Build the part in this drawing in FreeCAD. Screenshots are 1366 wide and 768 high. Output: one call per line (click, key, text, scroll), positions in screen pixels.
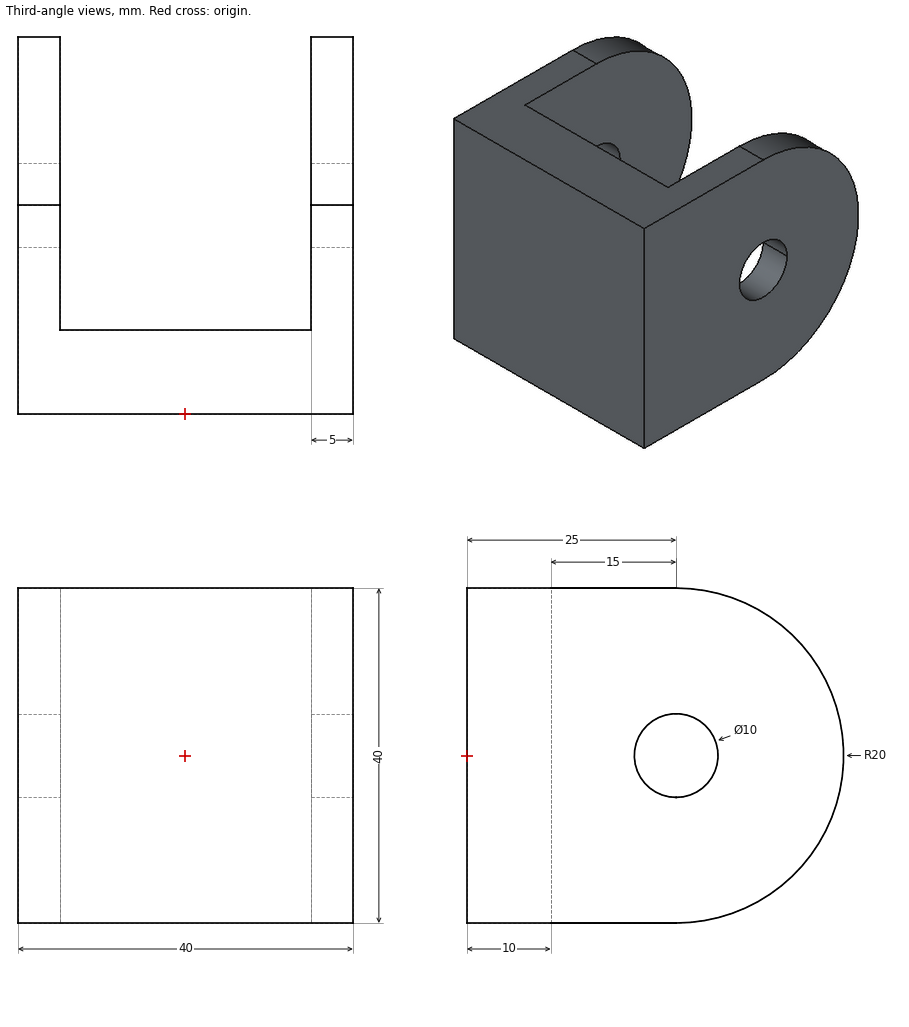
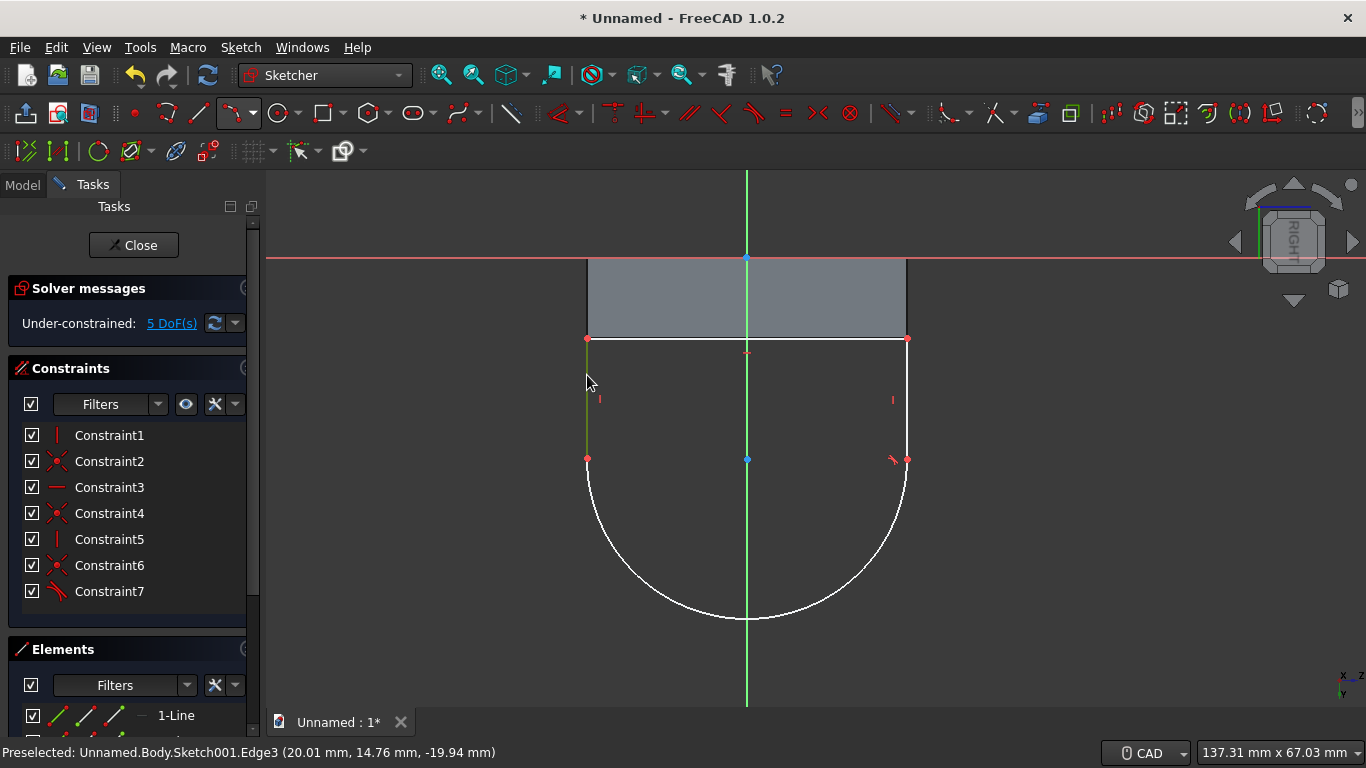
click(653, 588)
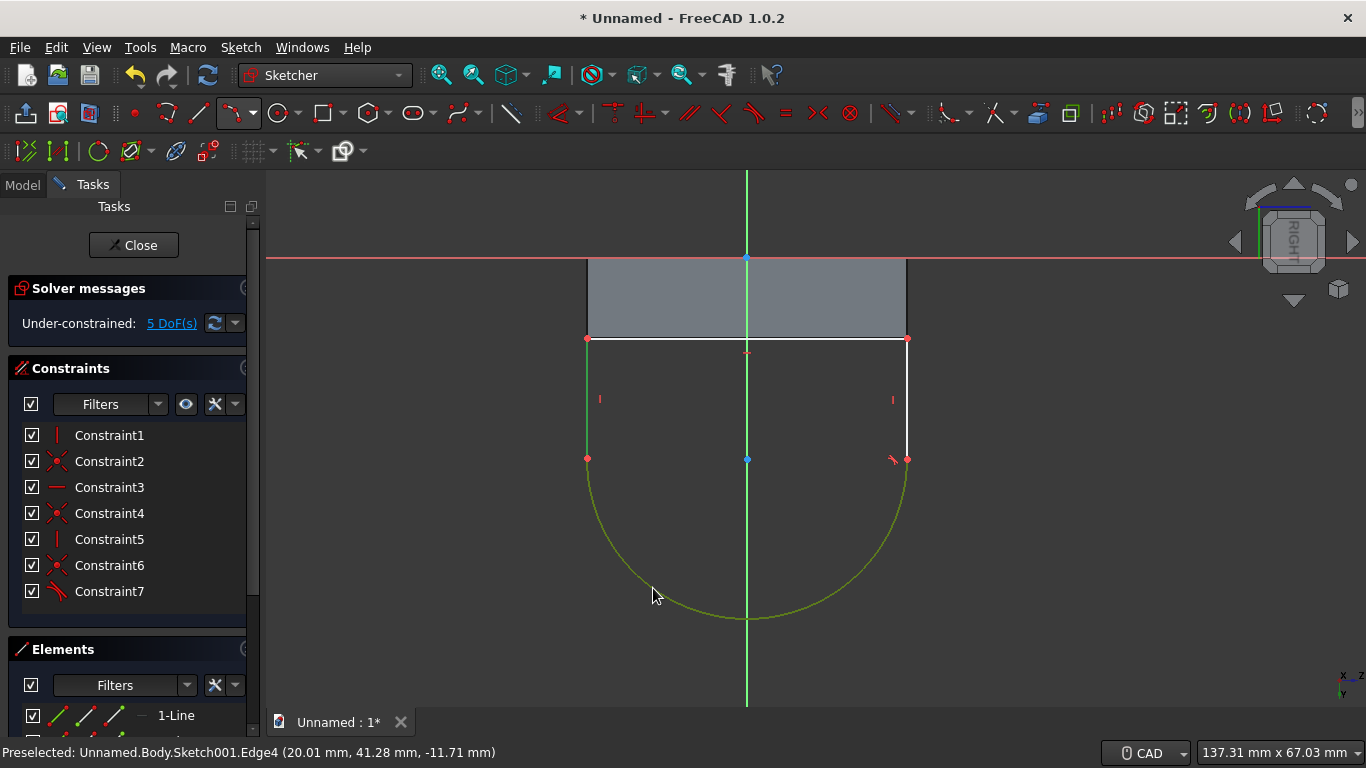
key(t)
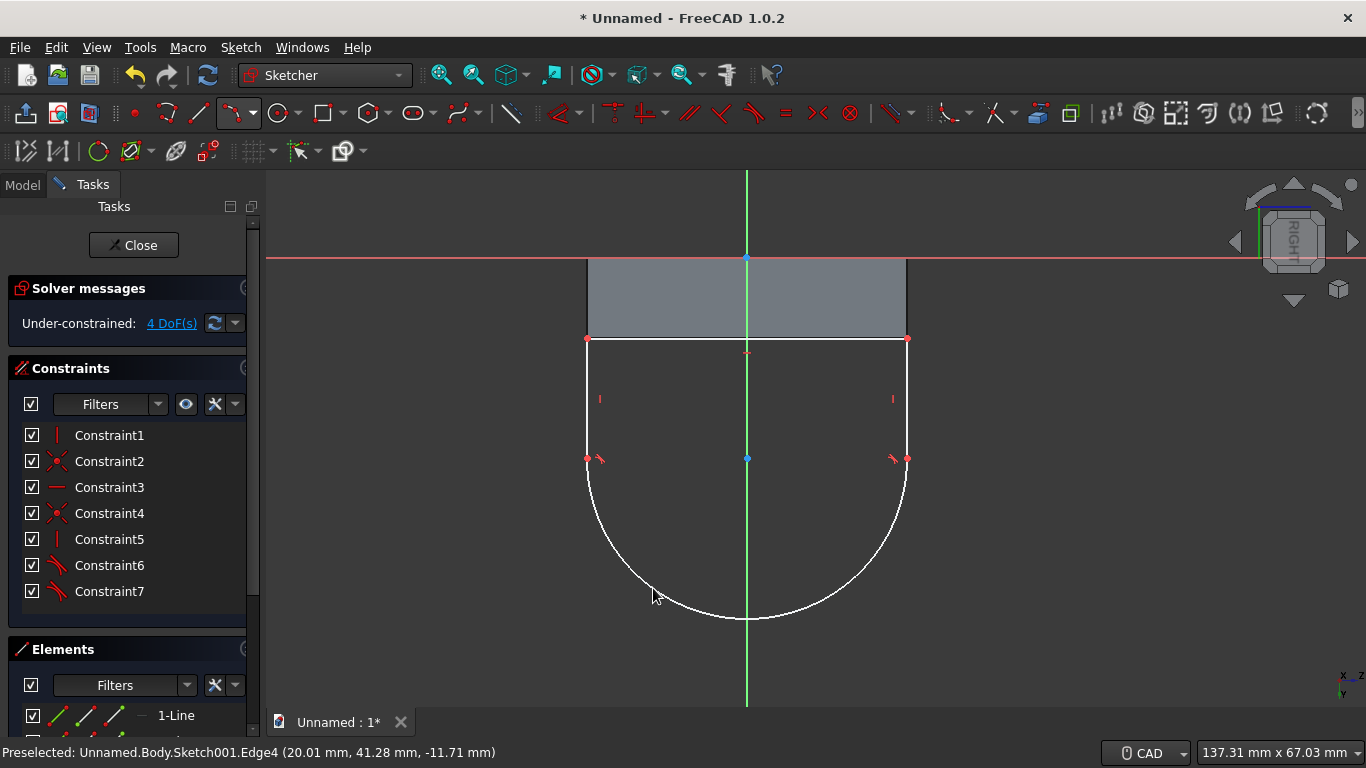
click(747, 459)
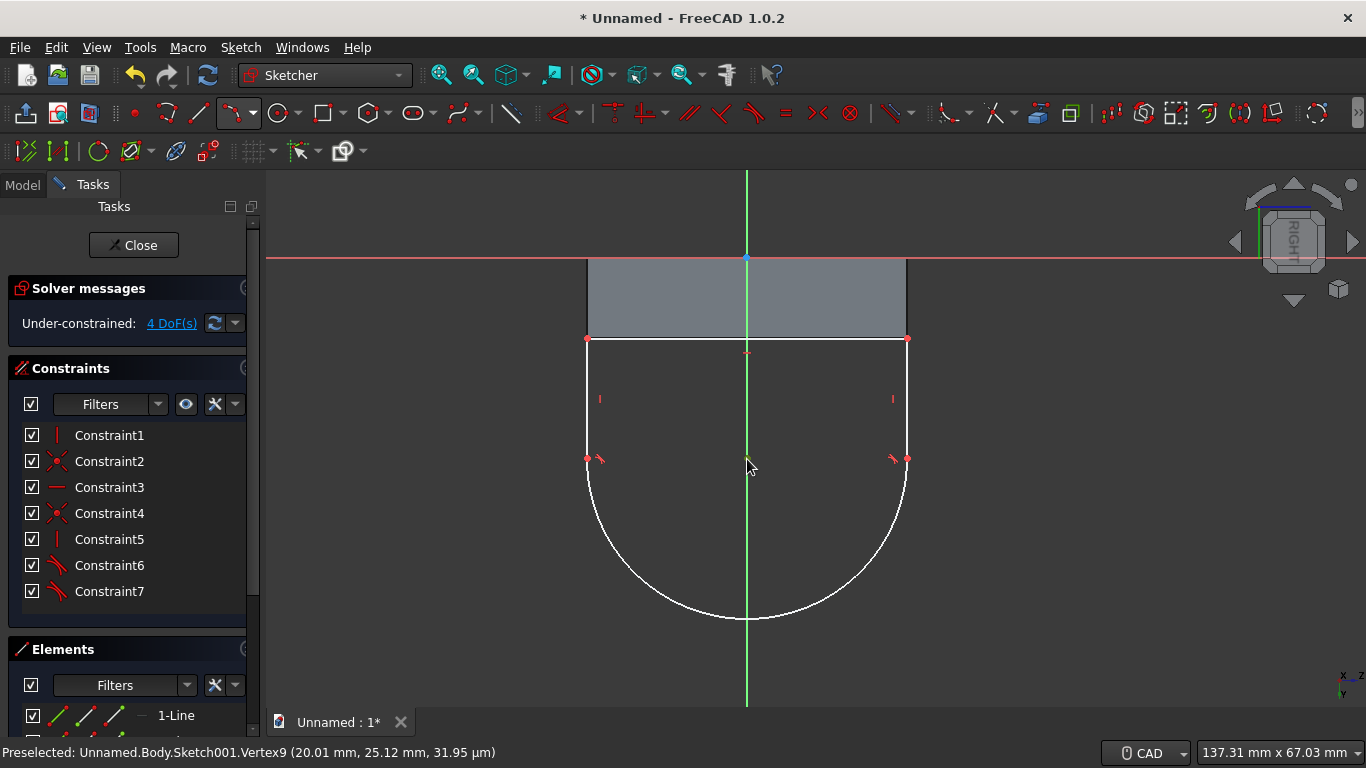
click(747, 576)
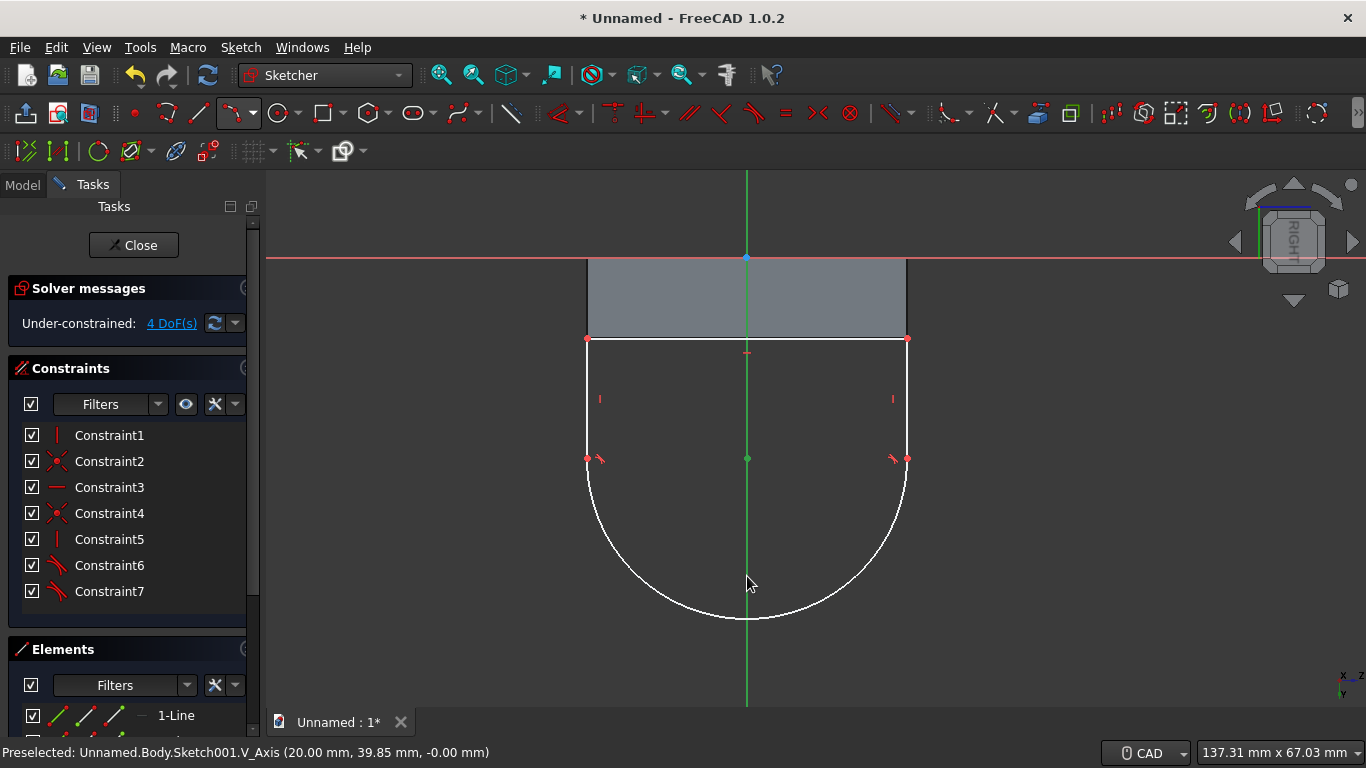
click(614, 114)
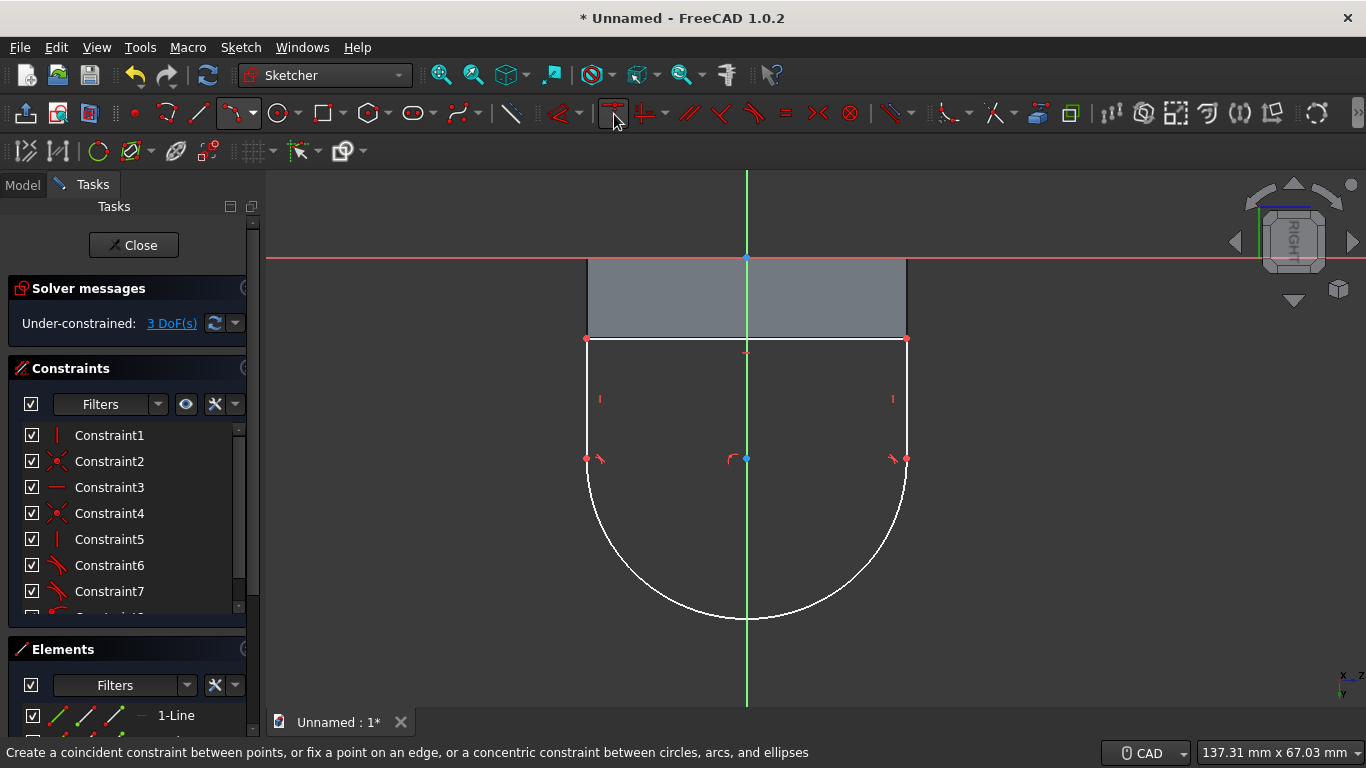
click(558, 114)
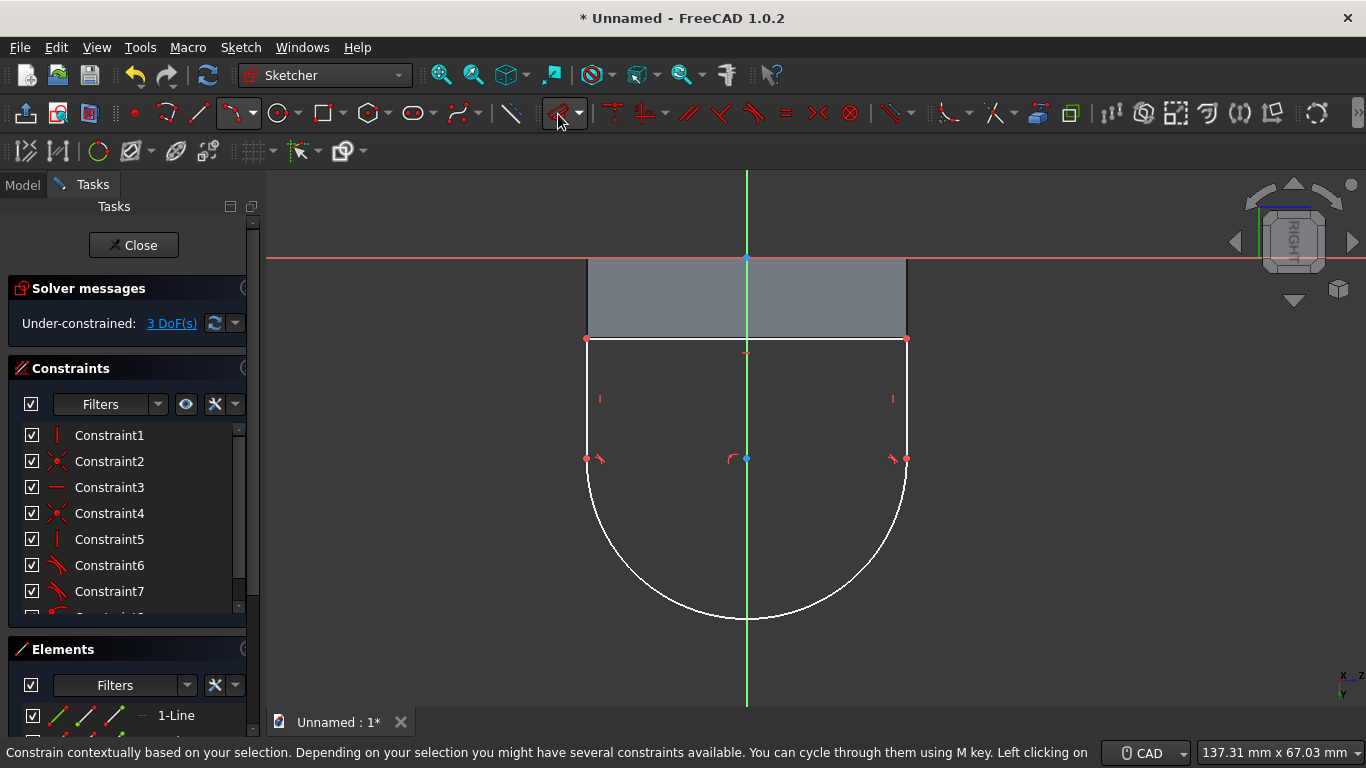
click(653, 588)
click(634, 614)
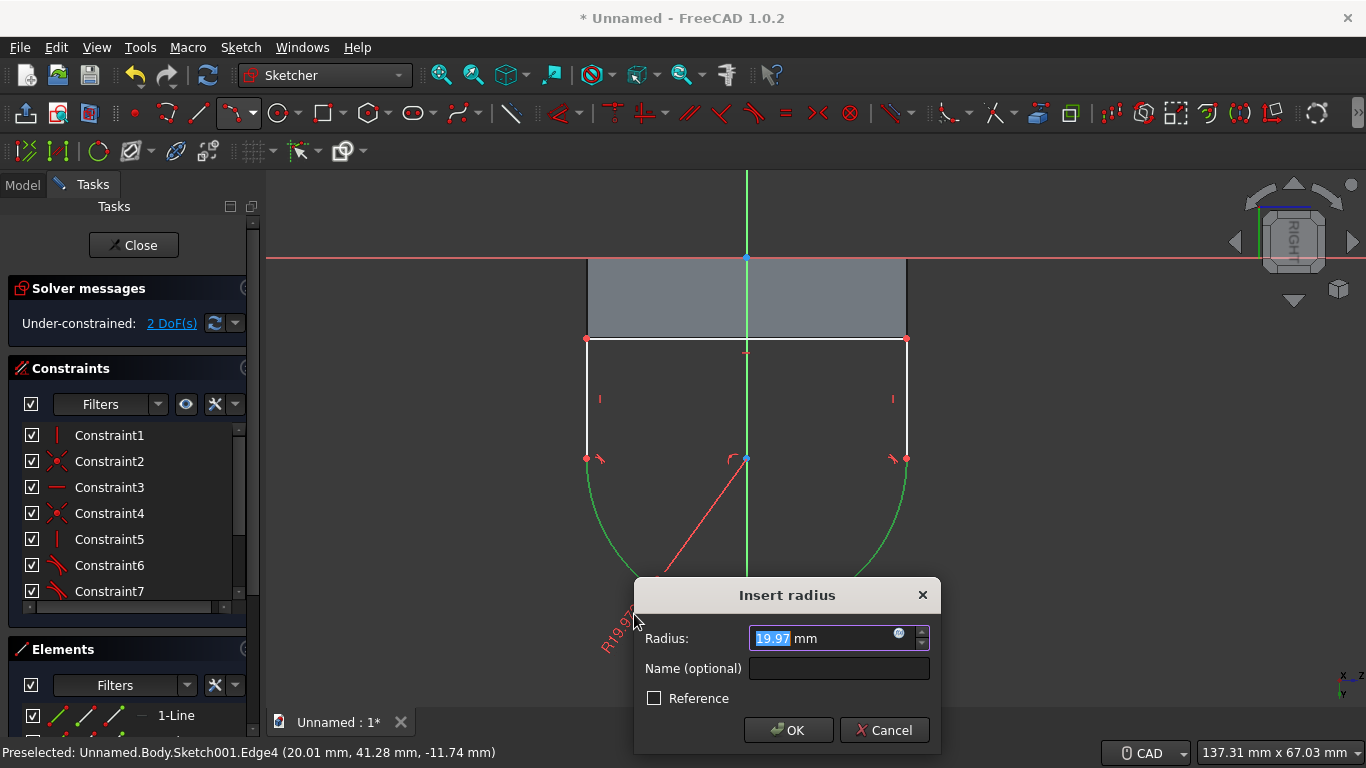
text(20)
key(Return)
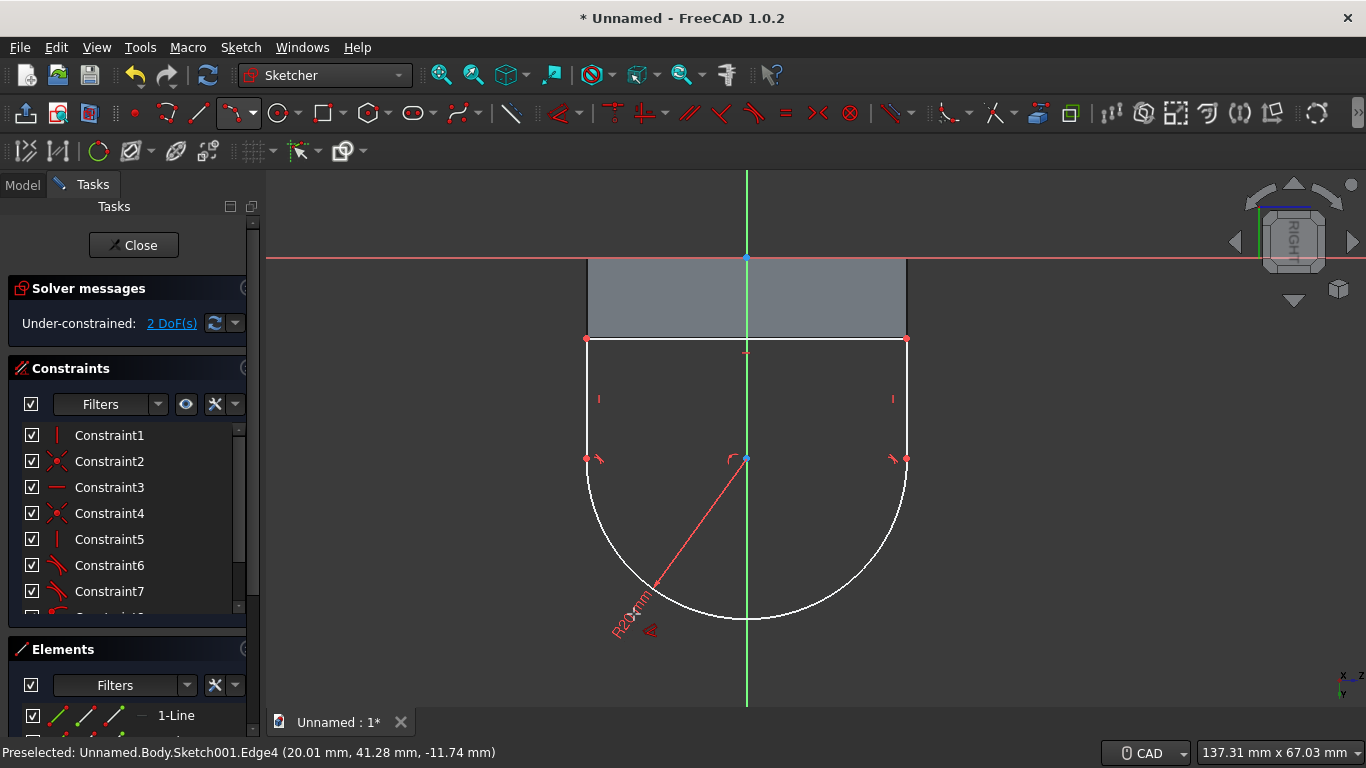
click(907, 423)
click(941, 399)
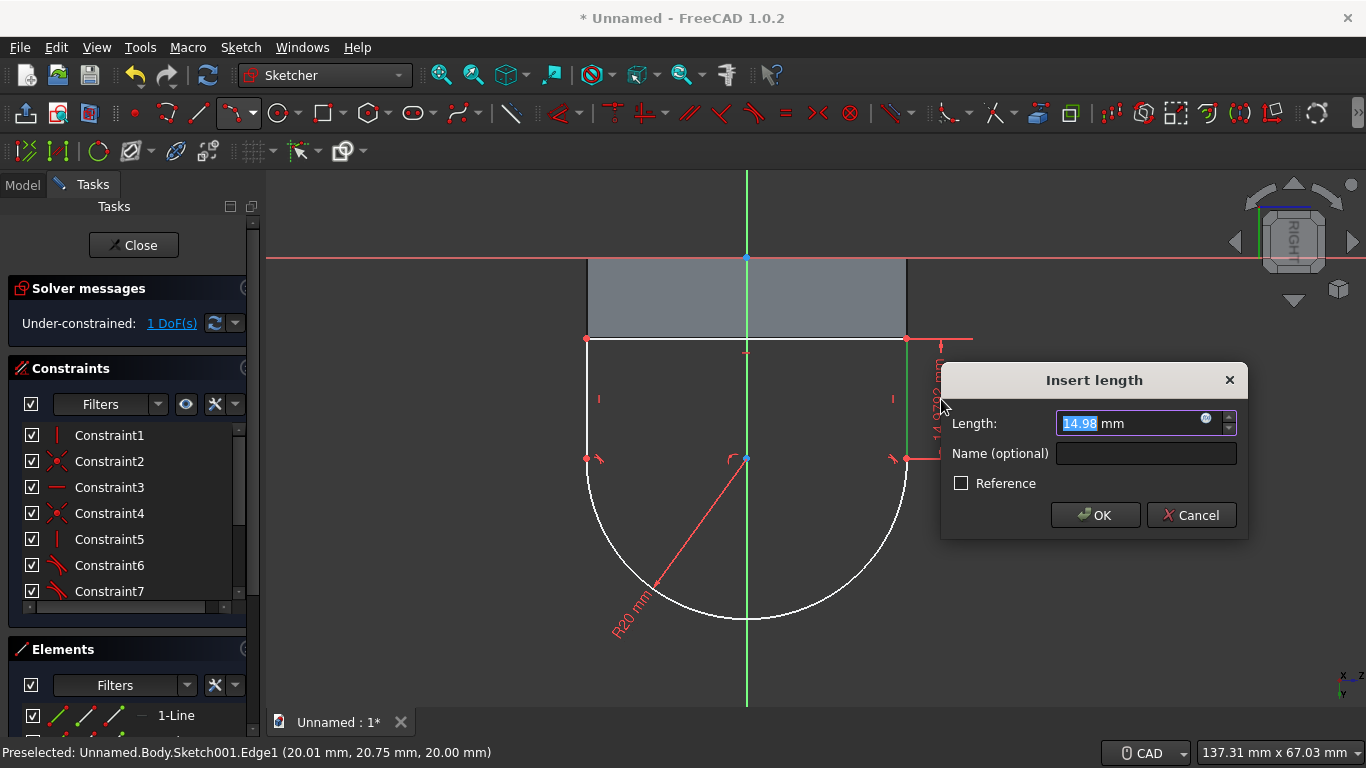
text(15)
key(Return)